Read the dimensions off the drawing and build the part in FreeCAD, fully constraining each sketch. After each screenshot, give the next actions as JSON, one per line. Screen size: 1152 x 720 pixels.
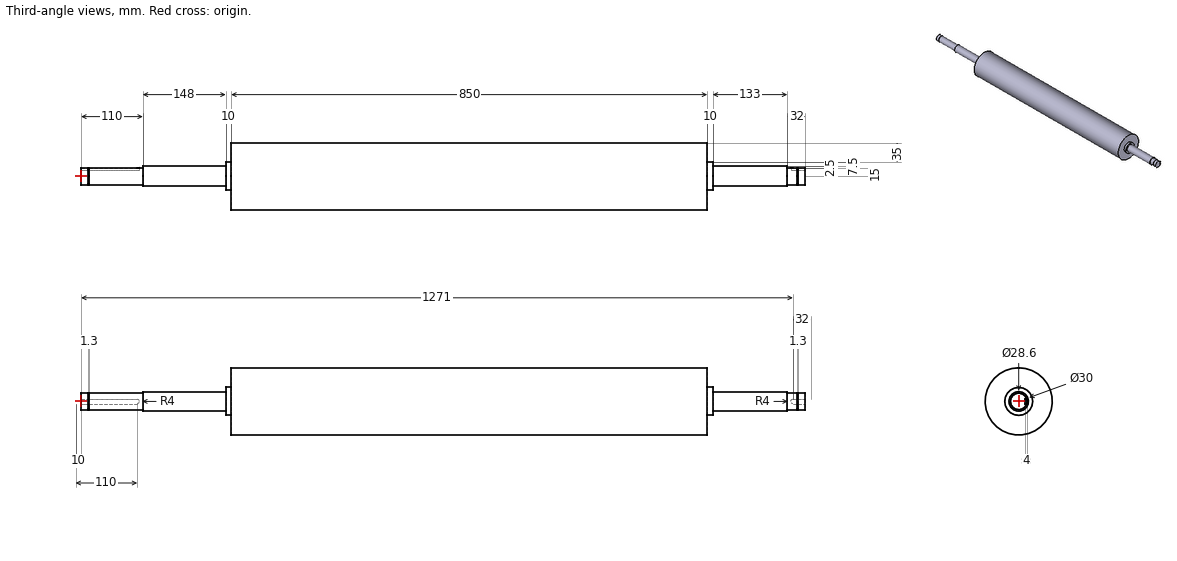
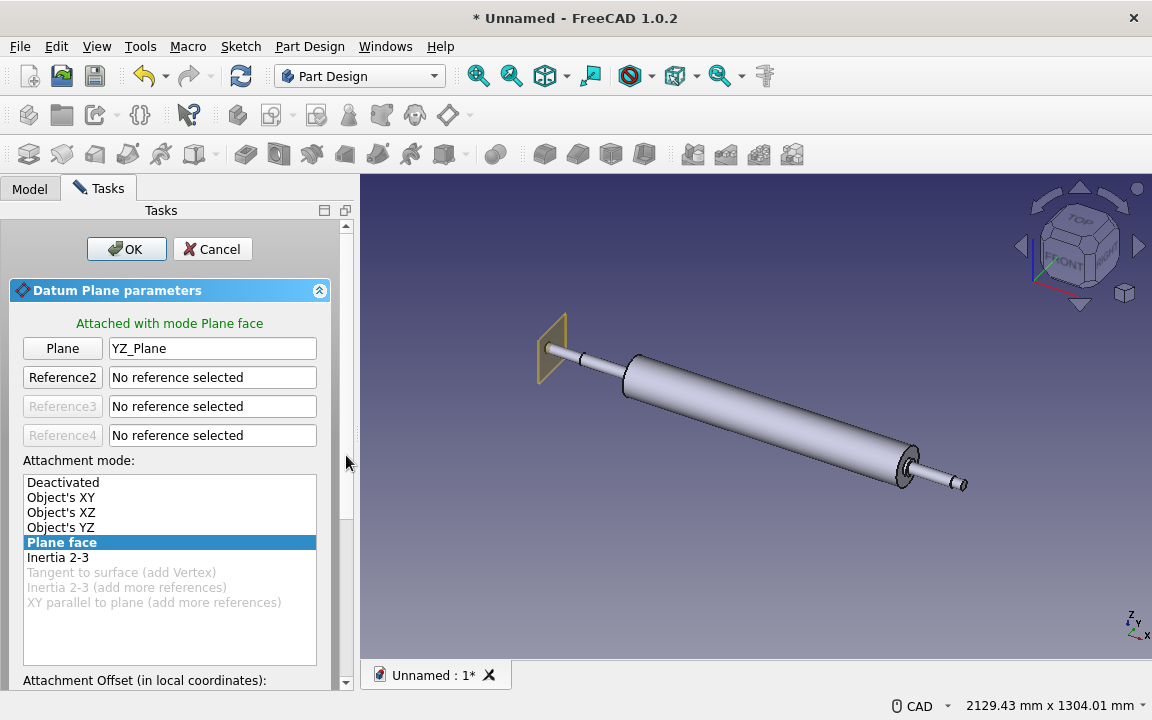
{"action": "left_click", "coordinate": [127, 249]}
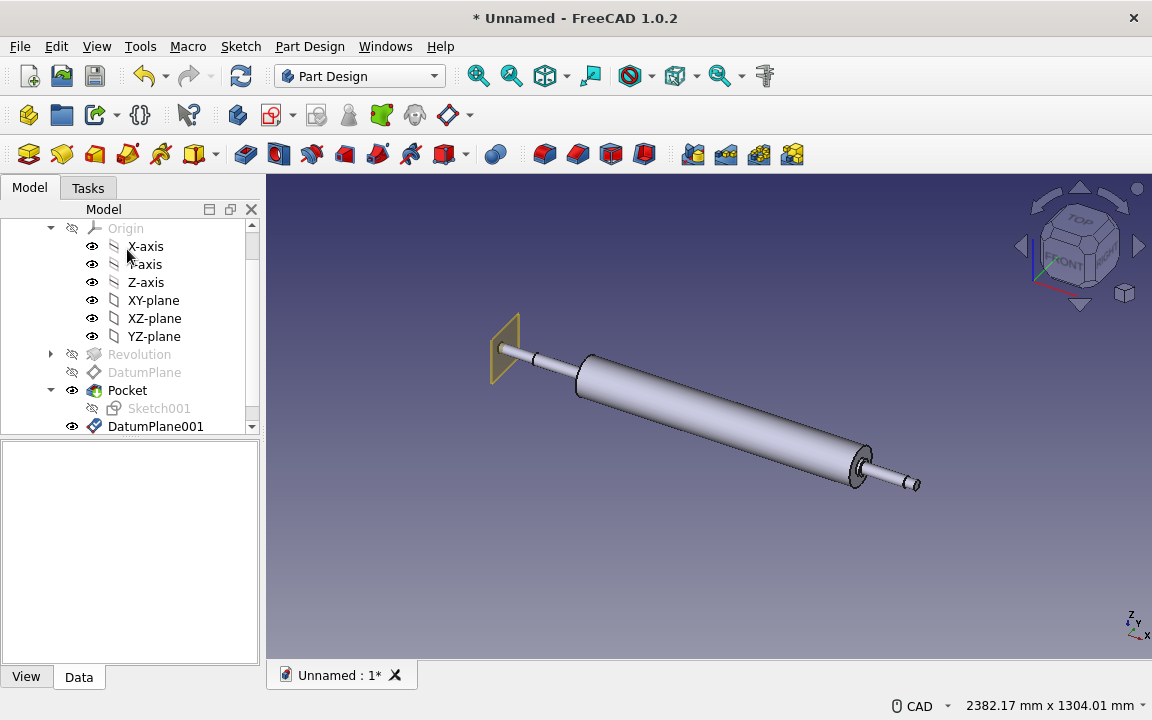
{"action": "left_click", "coordinate": [117, 426]}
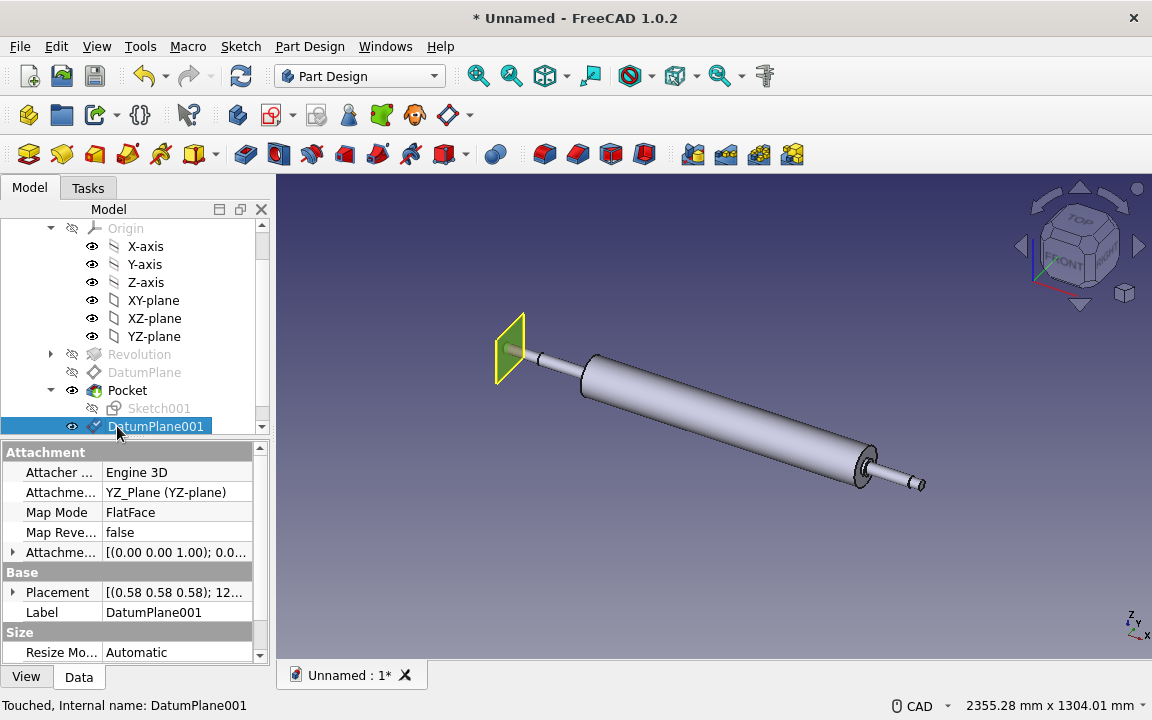
{"action": "left_click", "coordinate": [270, 116]}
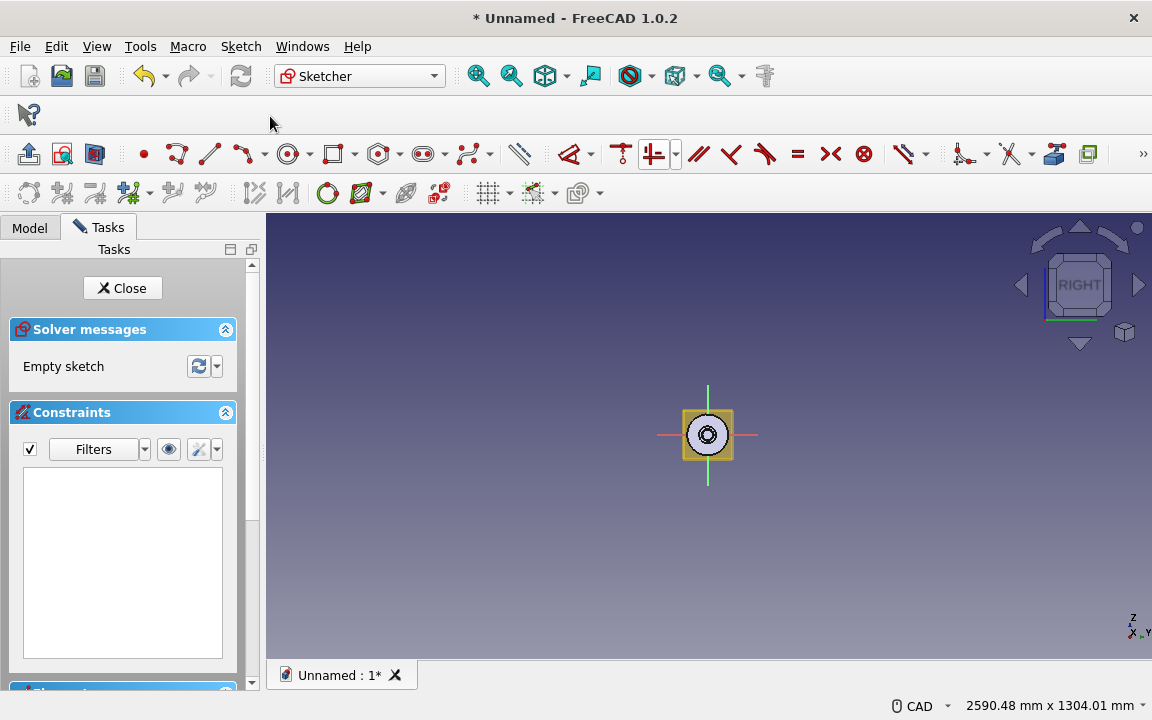
{"action": "left_click", "coordinate": [95, 154]}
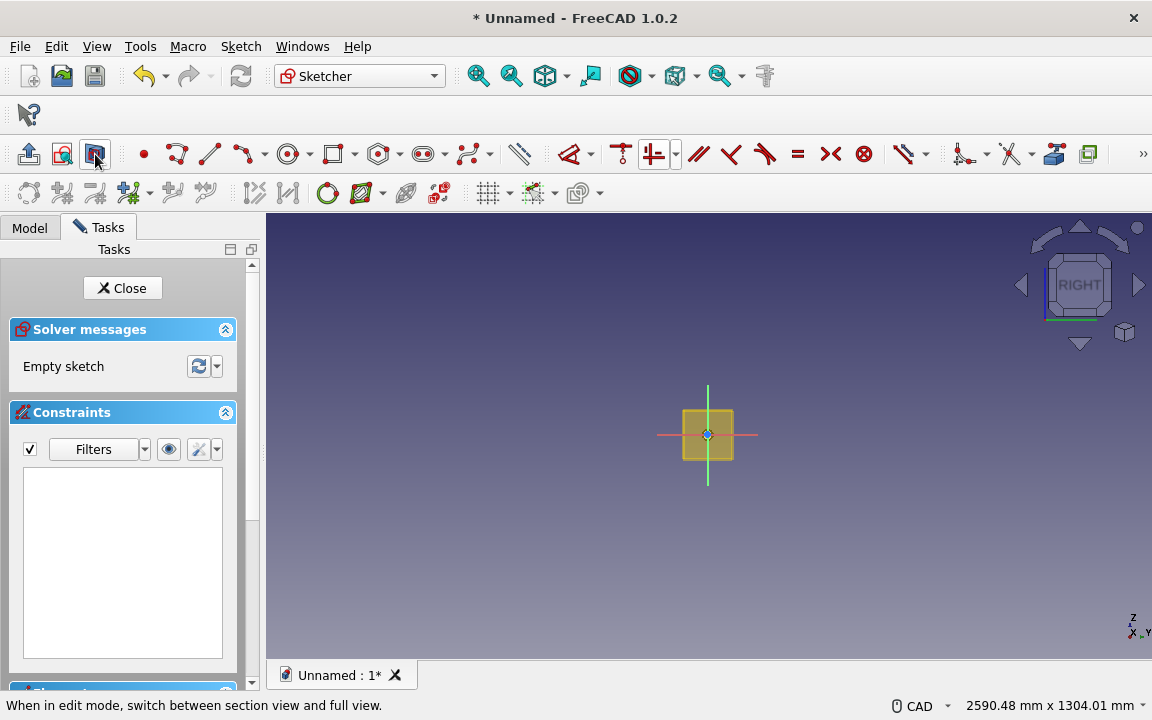
{"action": "scroll", "coordinate": [711, 435], "scroll_direction": "up", "scroll_amount": 15}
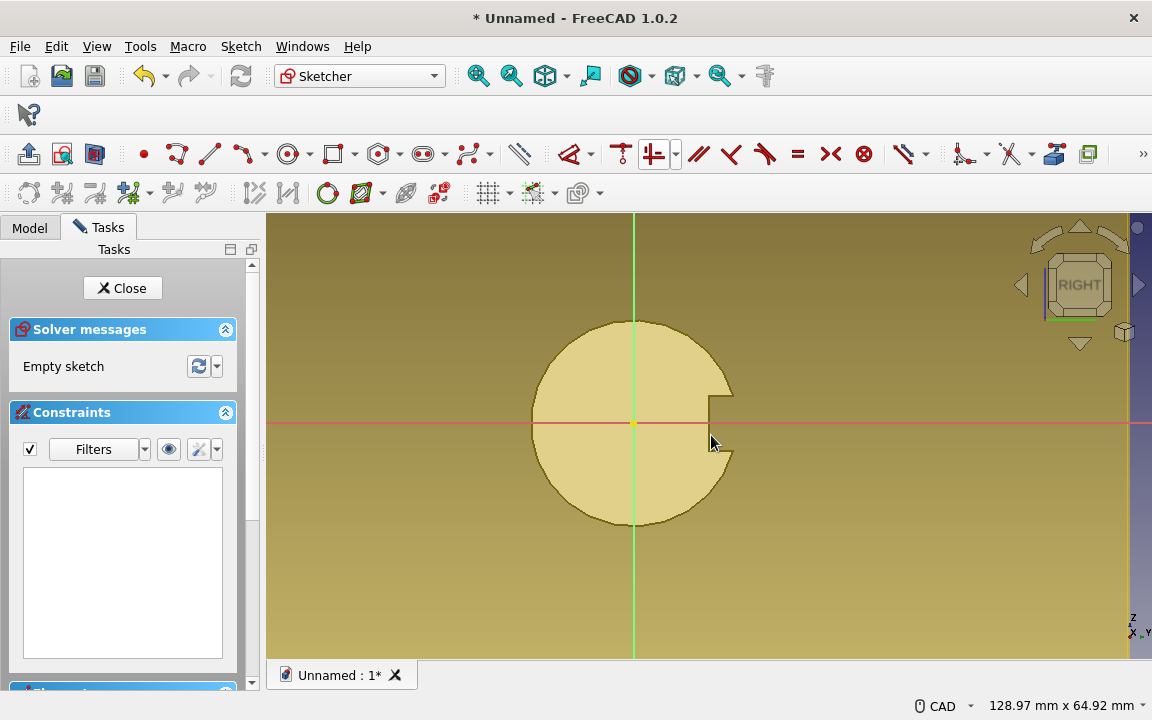
{"action": "key", "text": "g c"}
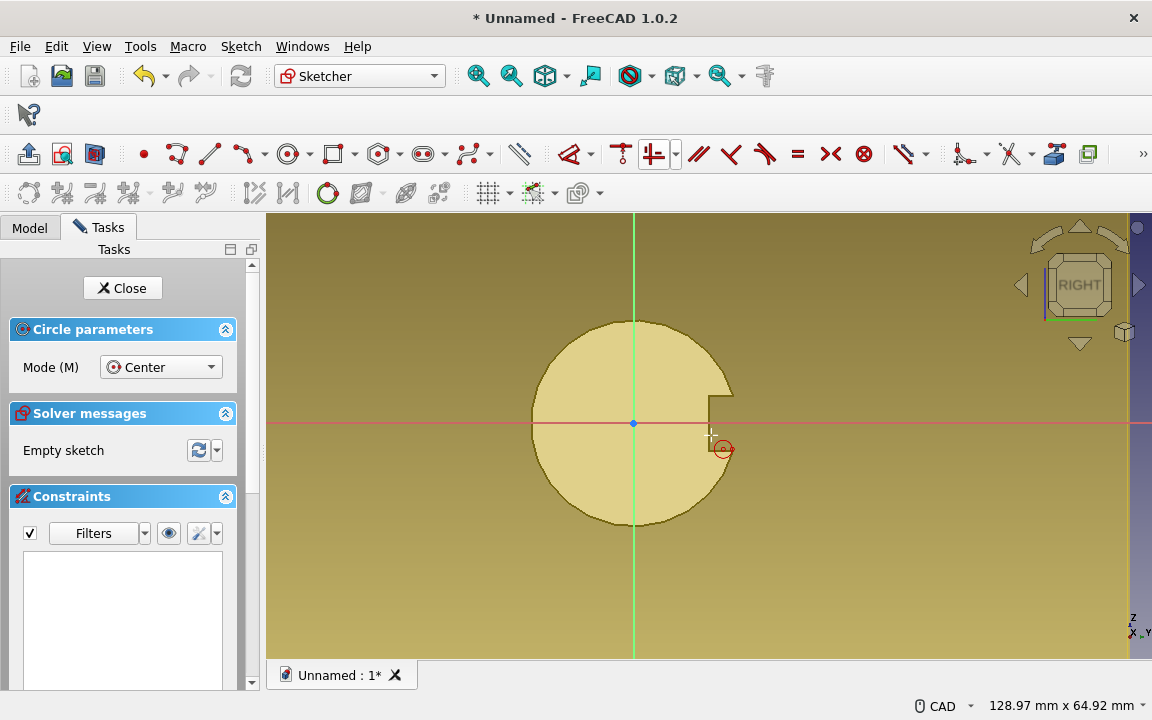
{"action": "left_click", "coordinate": [634, 423]}
{"action": "mouse_move", "coordinate": [707, 351]}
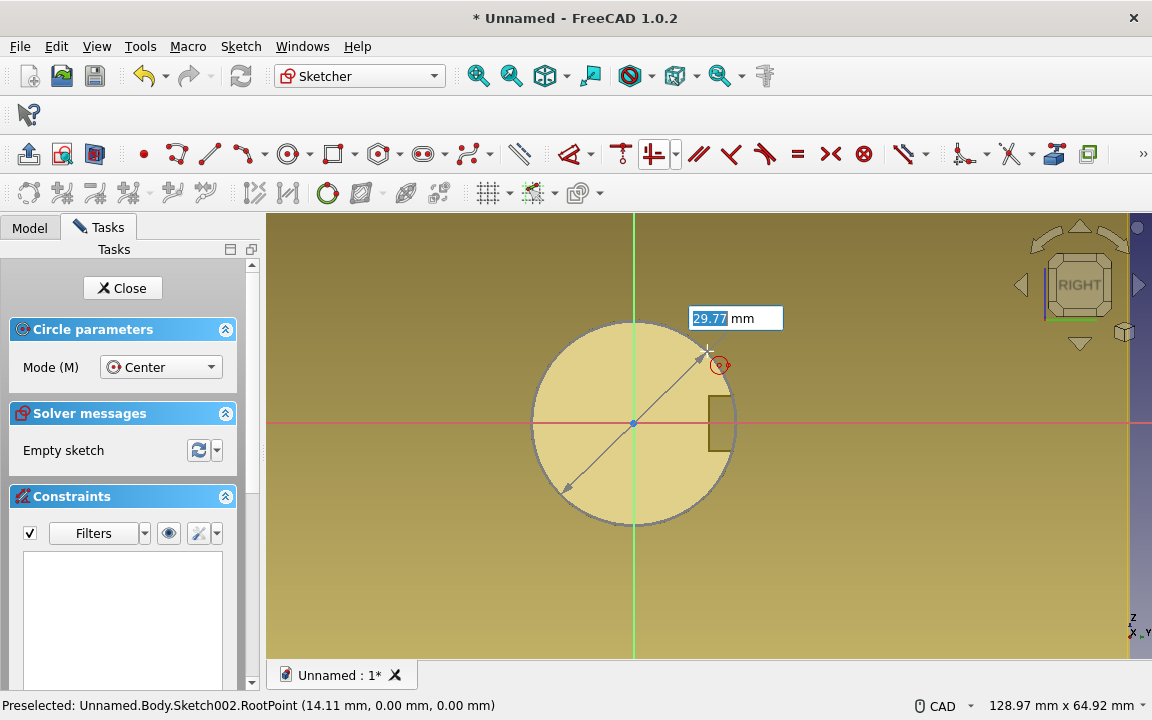
{"action": "type", "text": "30"}
{"action": "key", "text": "Return"}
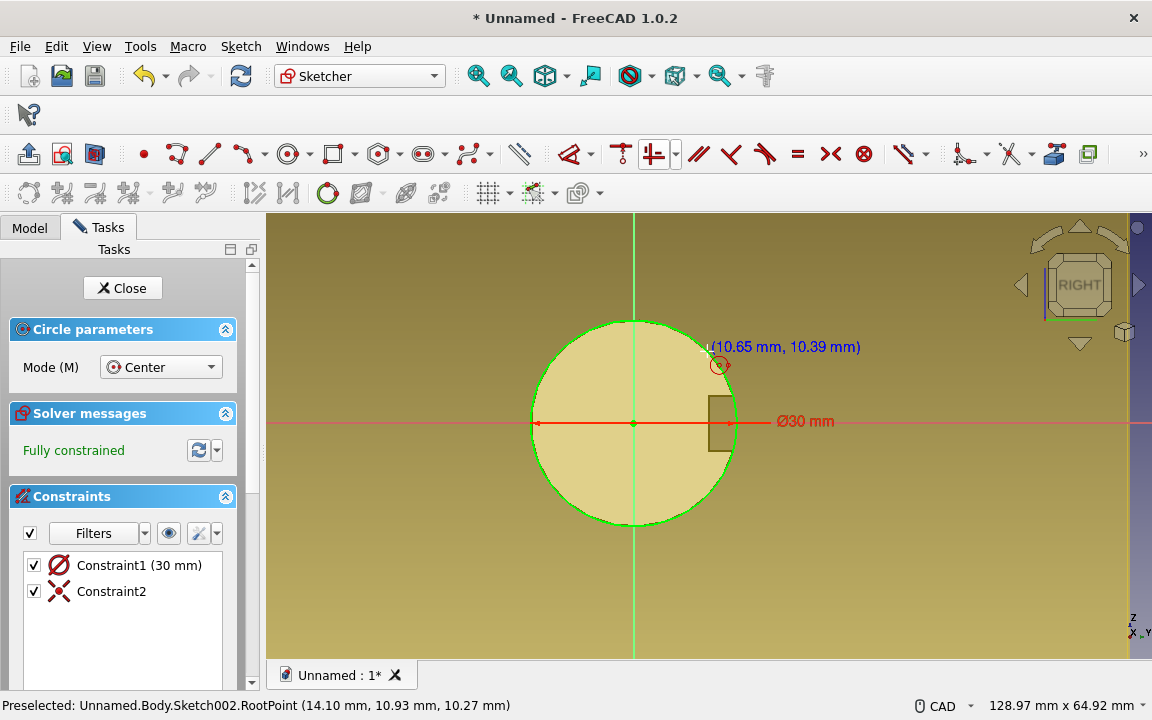
{"action": "left_click", "coordinate": [634, 423]}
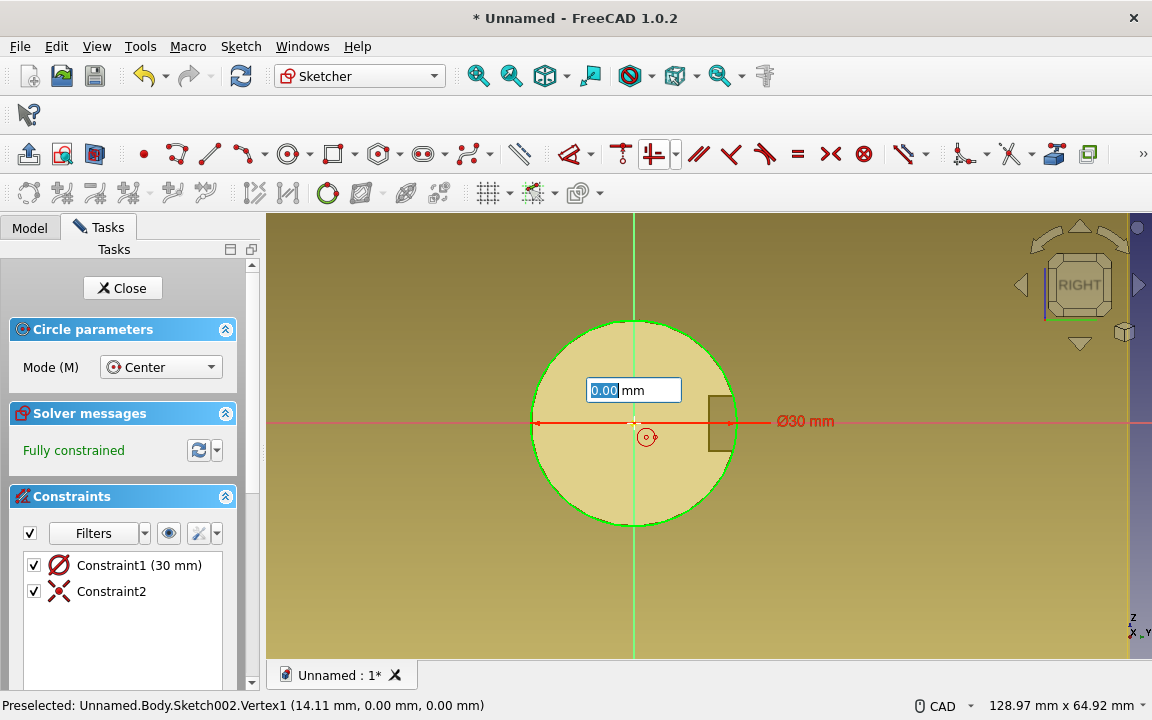
{"action": "scroll", "coordinate": [667, 331], "scroll_direction": "up", "scroll_amount": 6}
{"action": "mouse_move", "coordinate": [667, 331]}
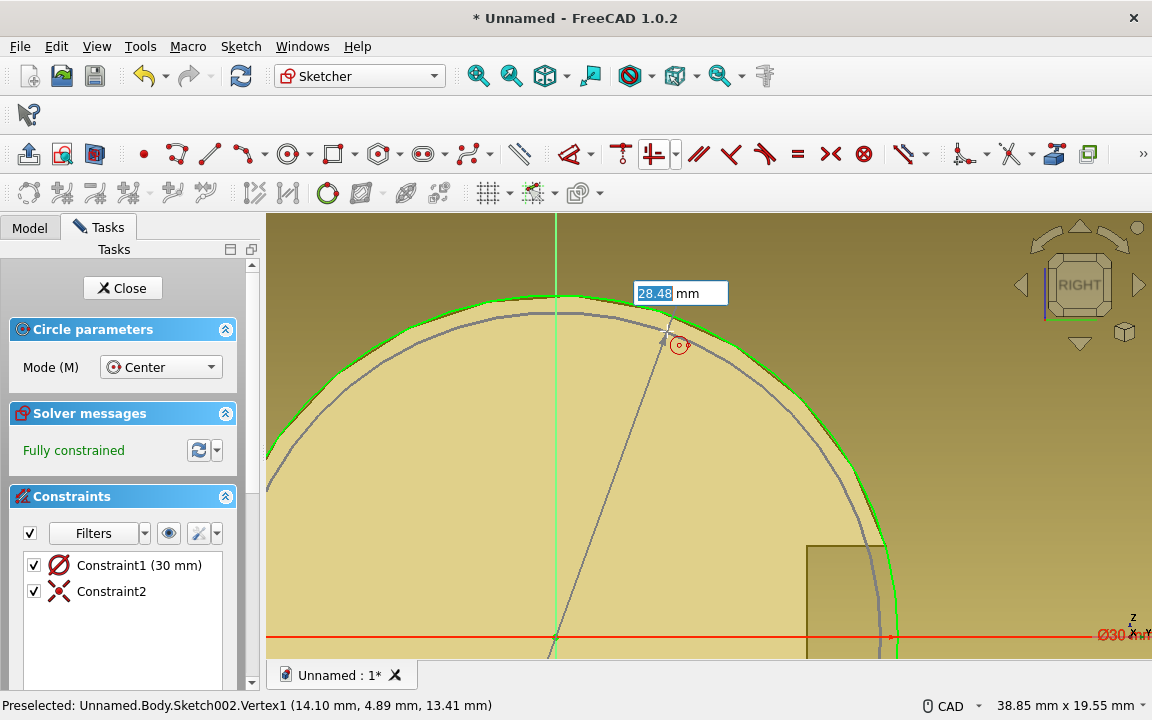
{"action": "type", "text": "28.6"}
{"action": "key", "text": "Return"}
{"action": "key", "text": "Escape"}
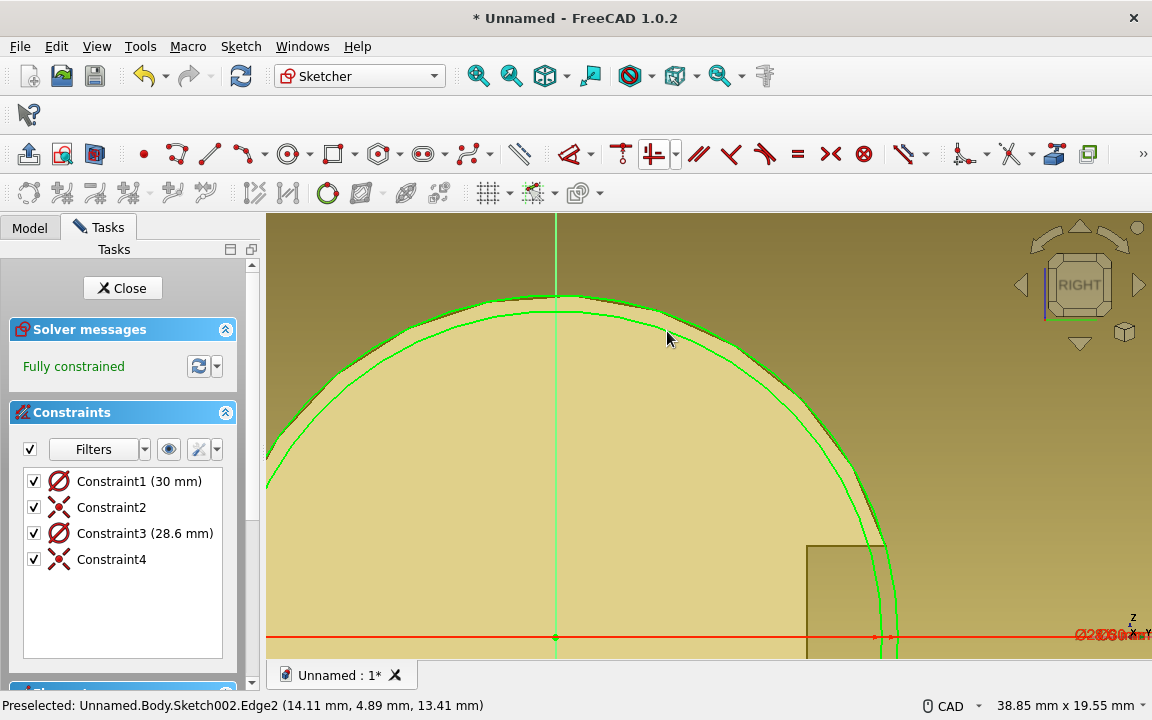
{"action": "left_click", "coordinate": [123, 288]}